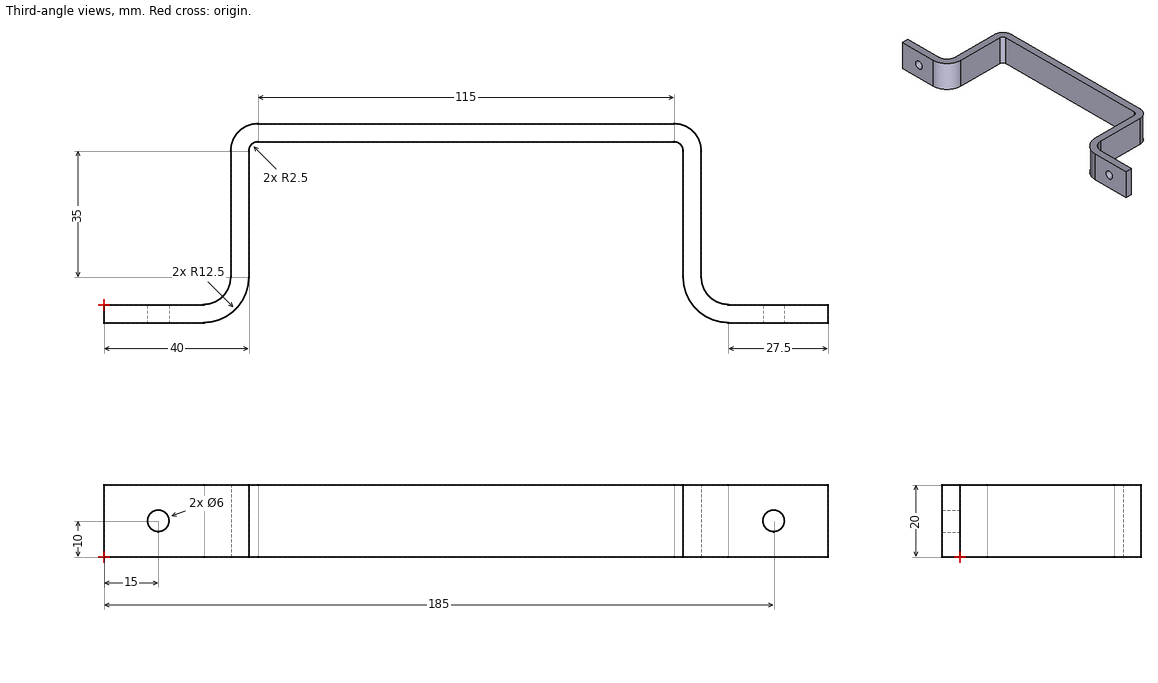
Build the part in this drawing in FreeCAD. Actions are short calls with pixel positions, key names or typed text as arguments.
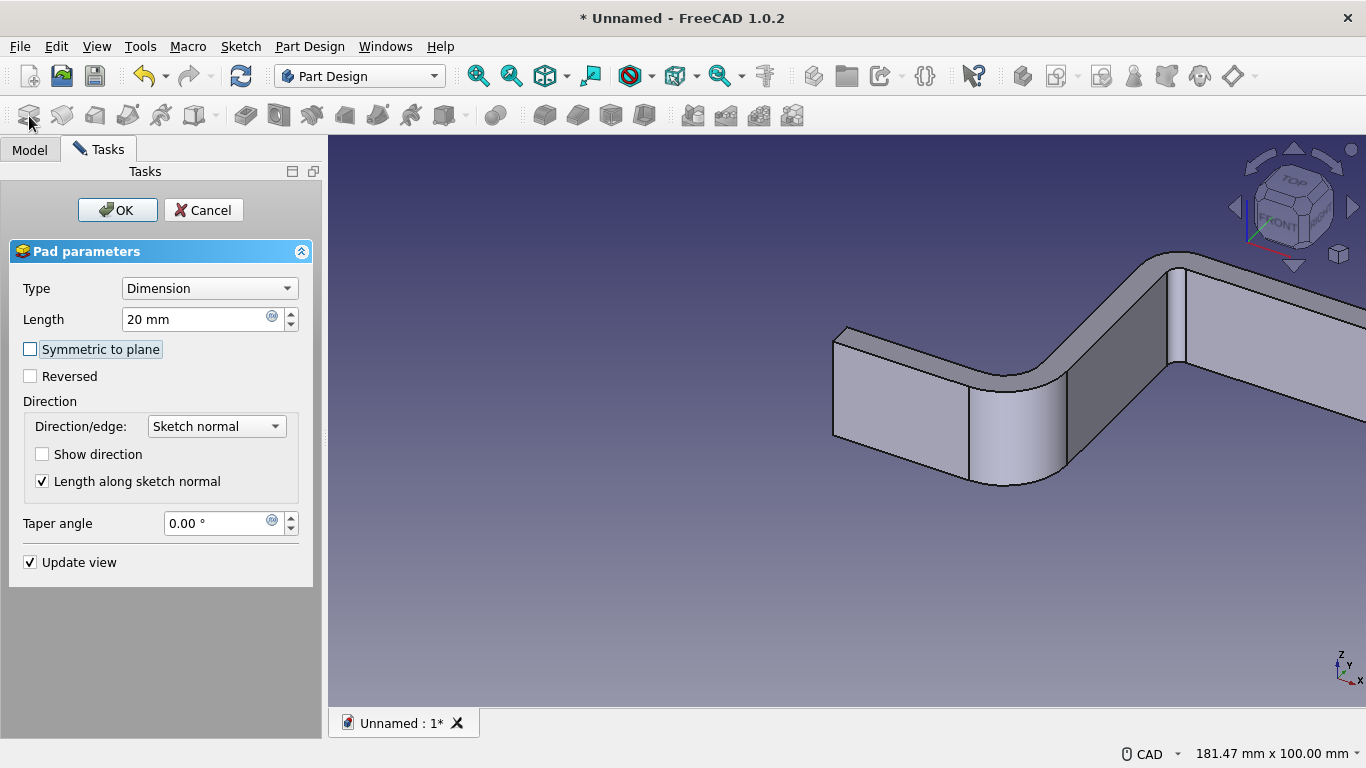
click(118, 210)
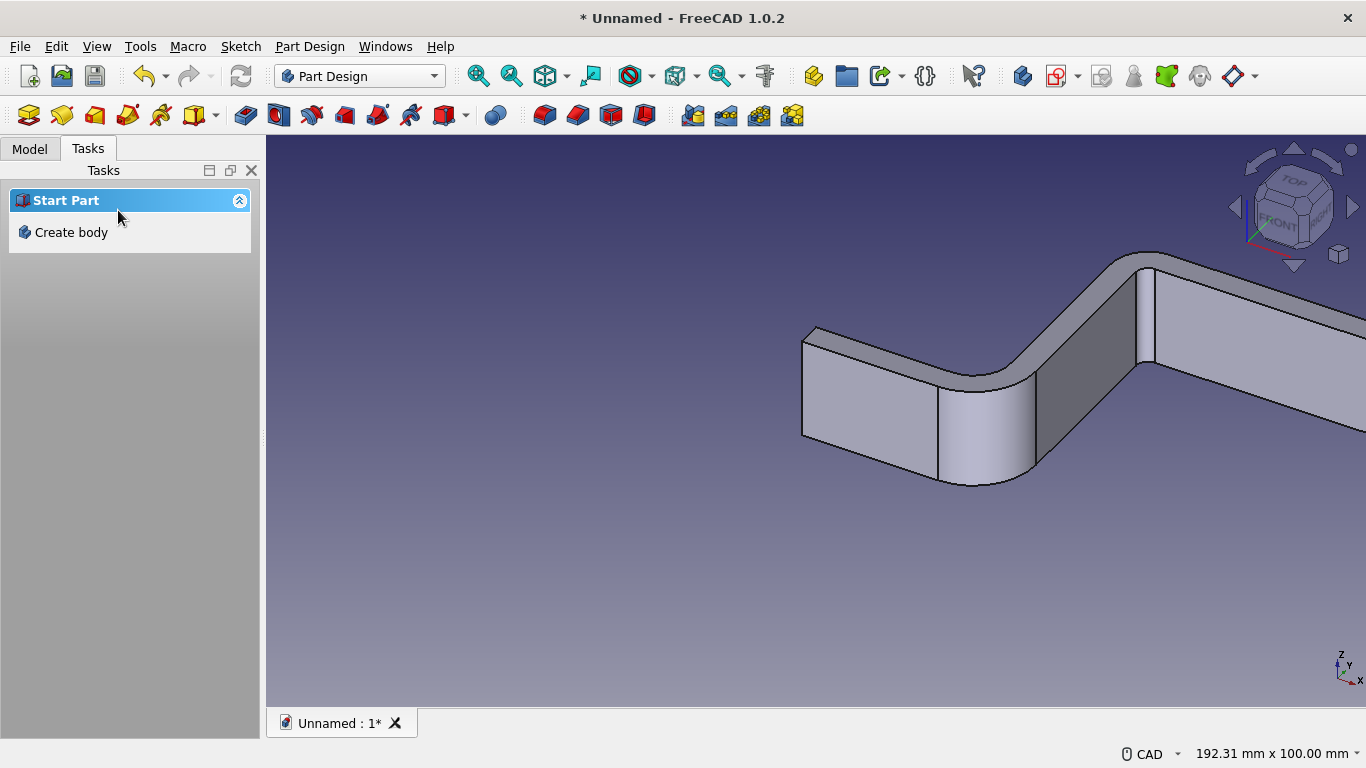
key(v)
key(f)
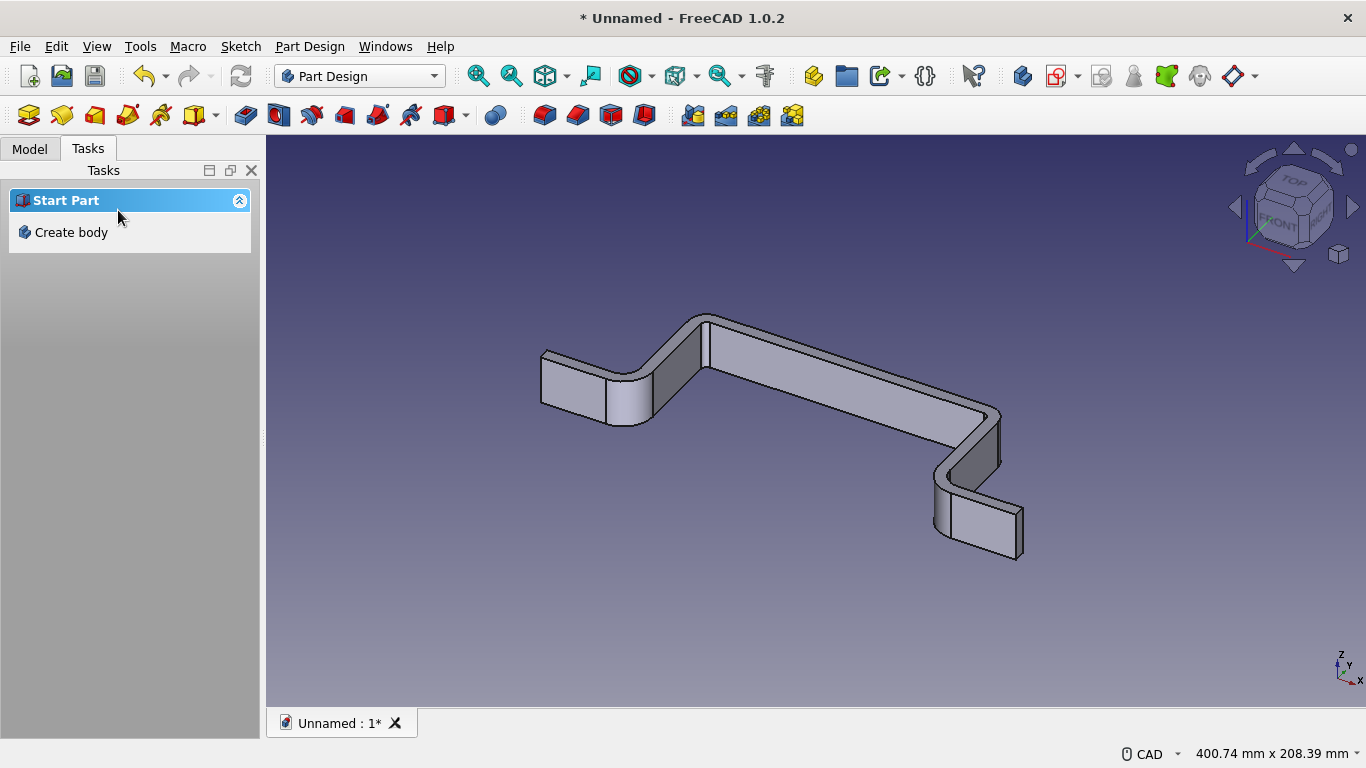
click(573, 390)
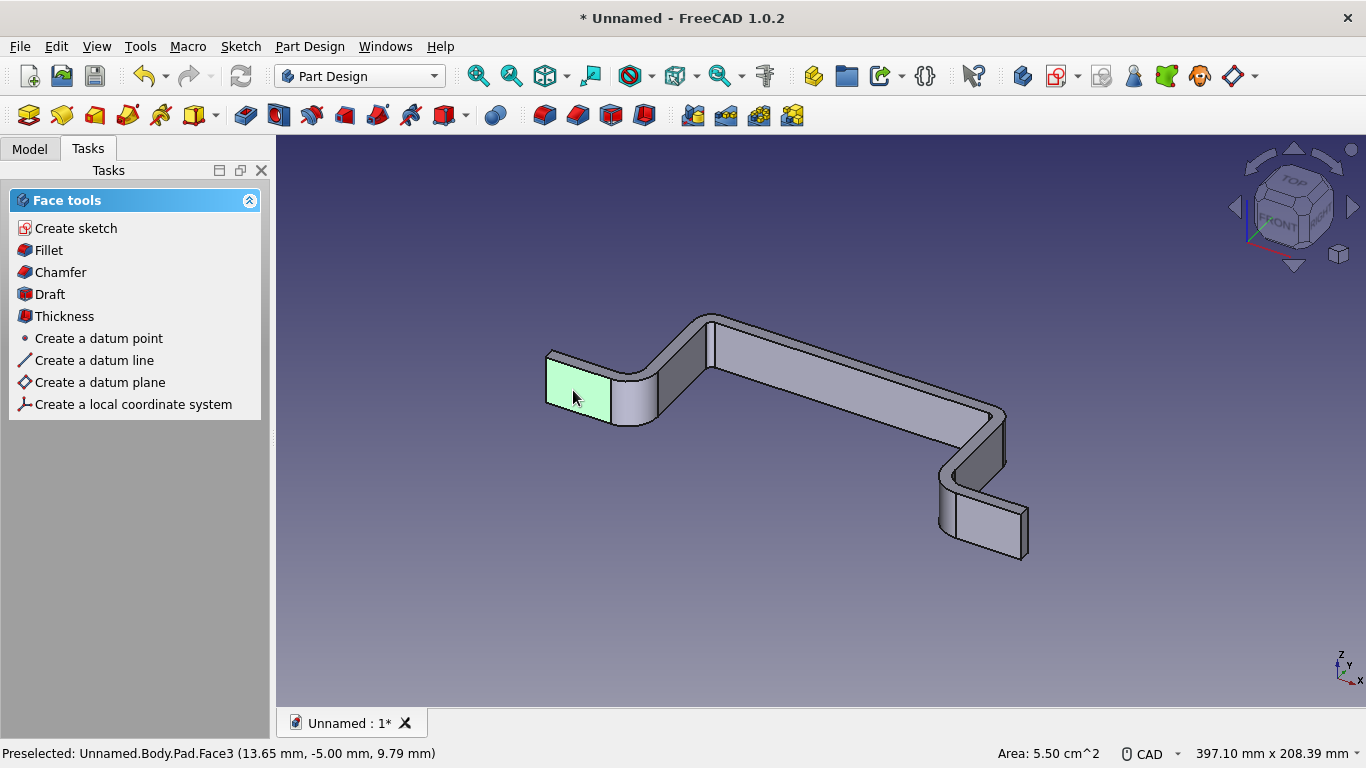
click(1056, 76)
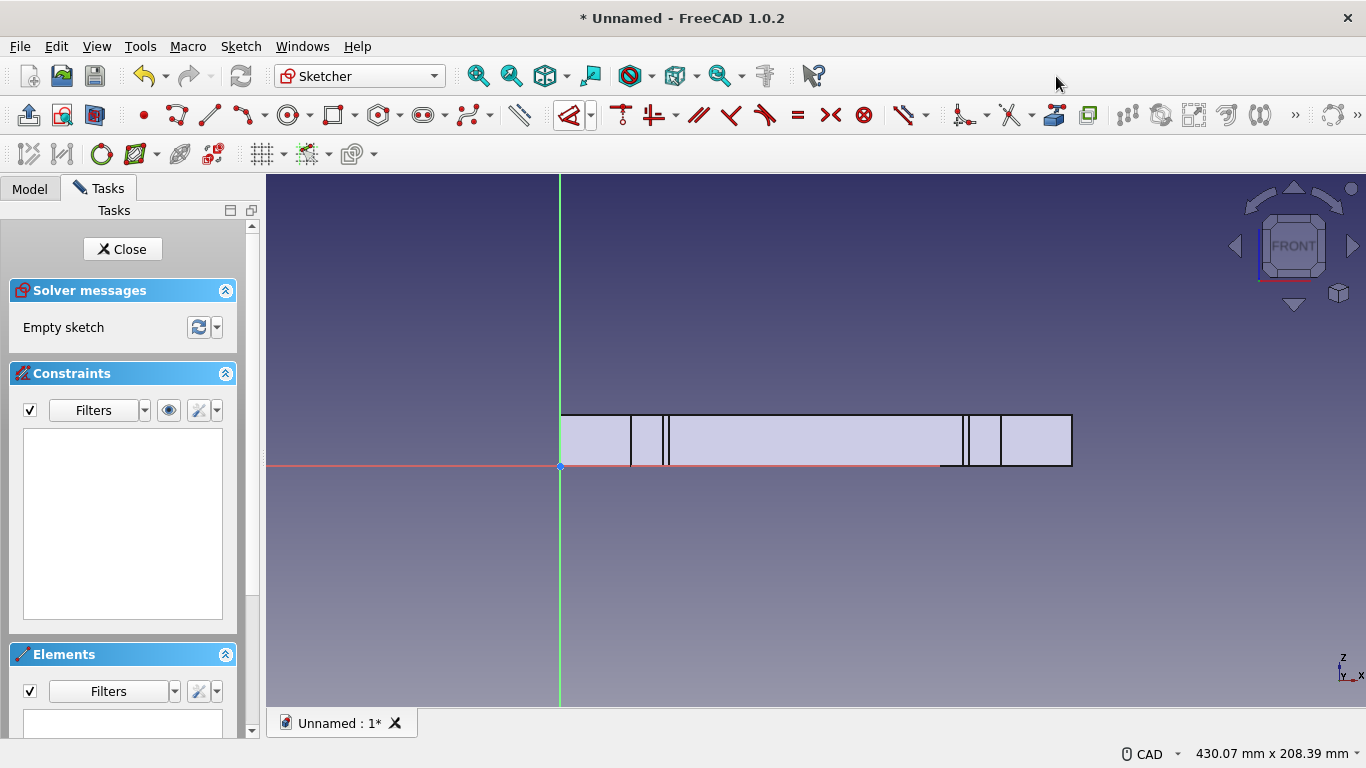
click(288, 116)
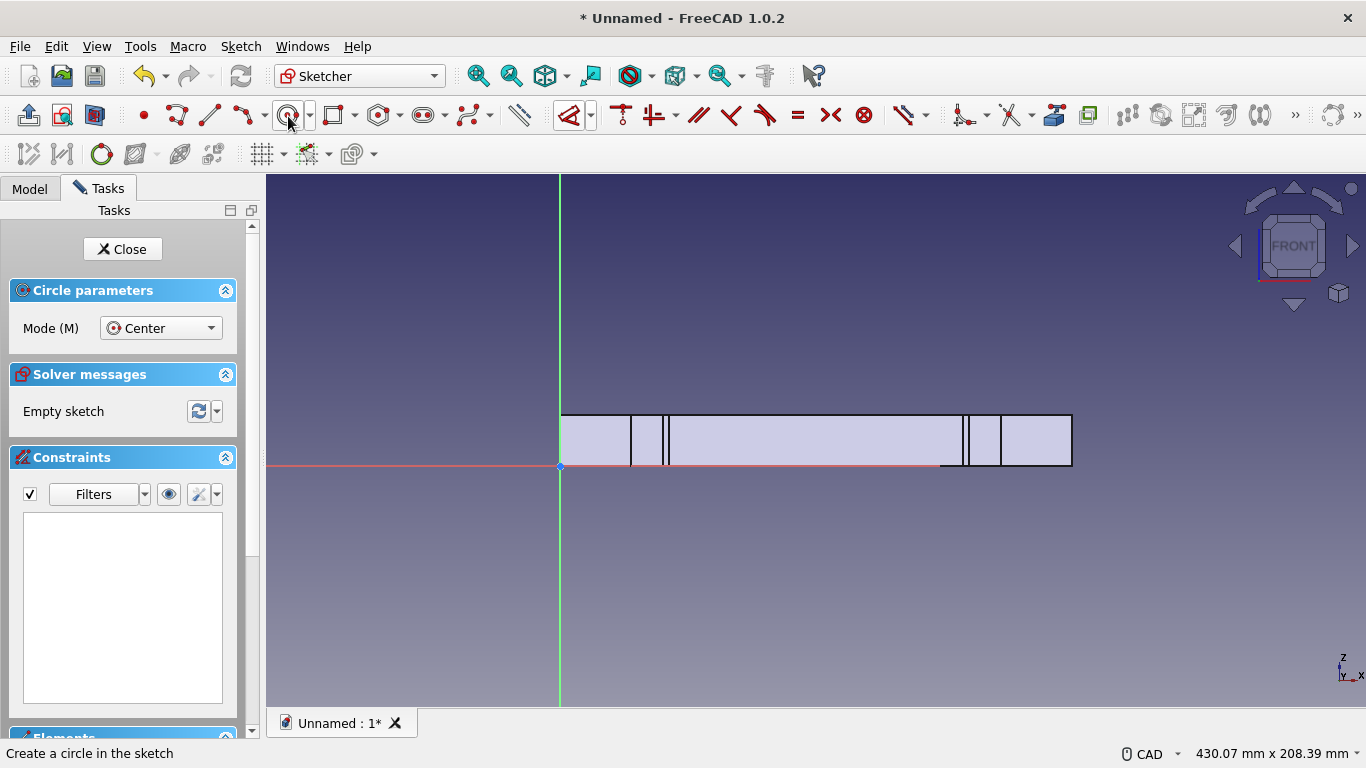
scroll(599, 440, up, 6)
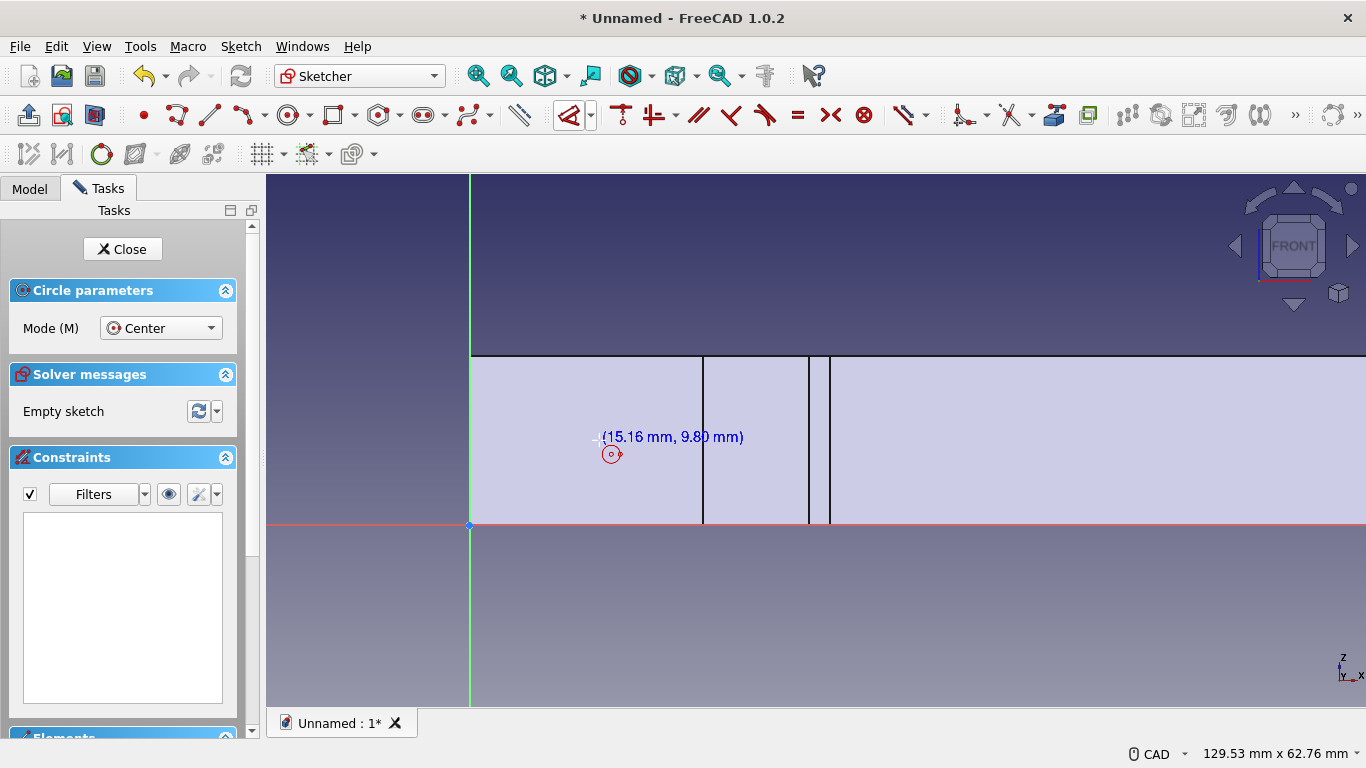
click(597, 440)
click(615, 422)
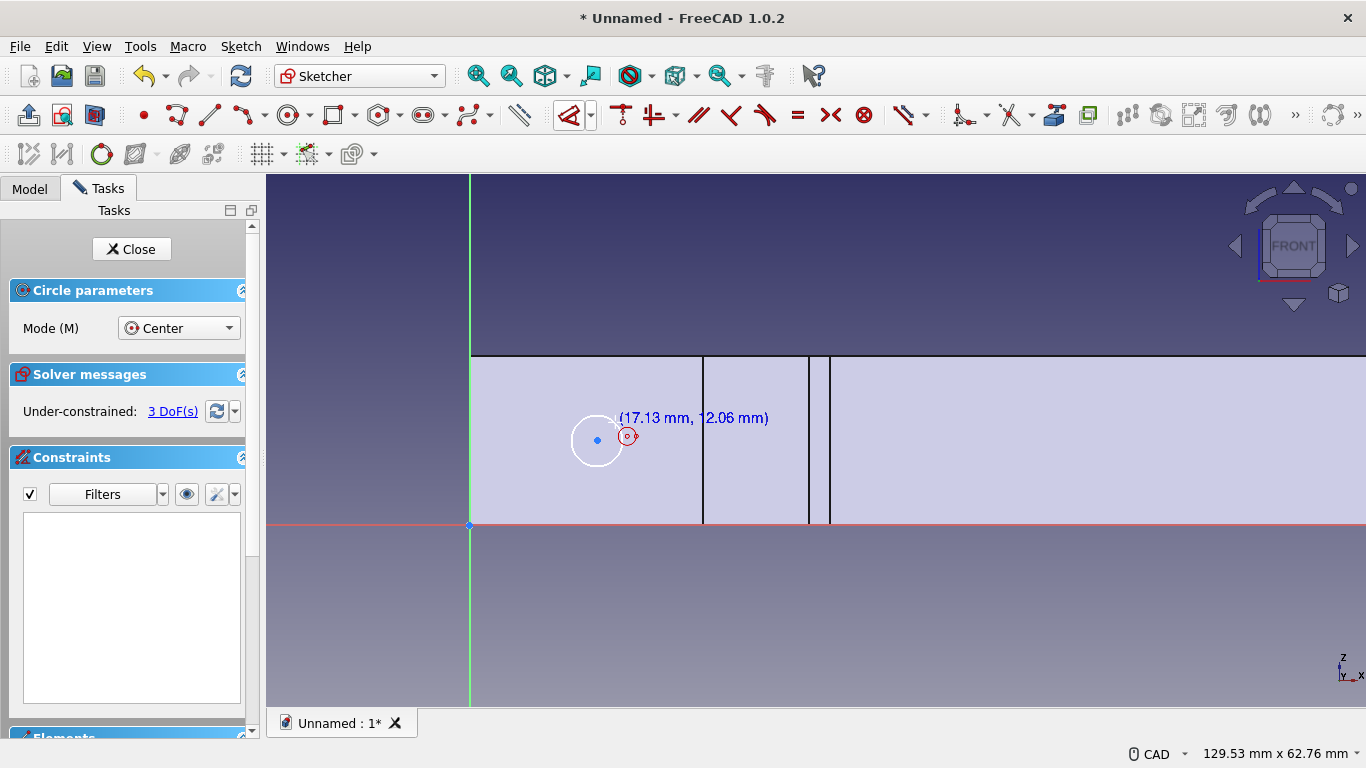
scroll(445, 423, down, 5)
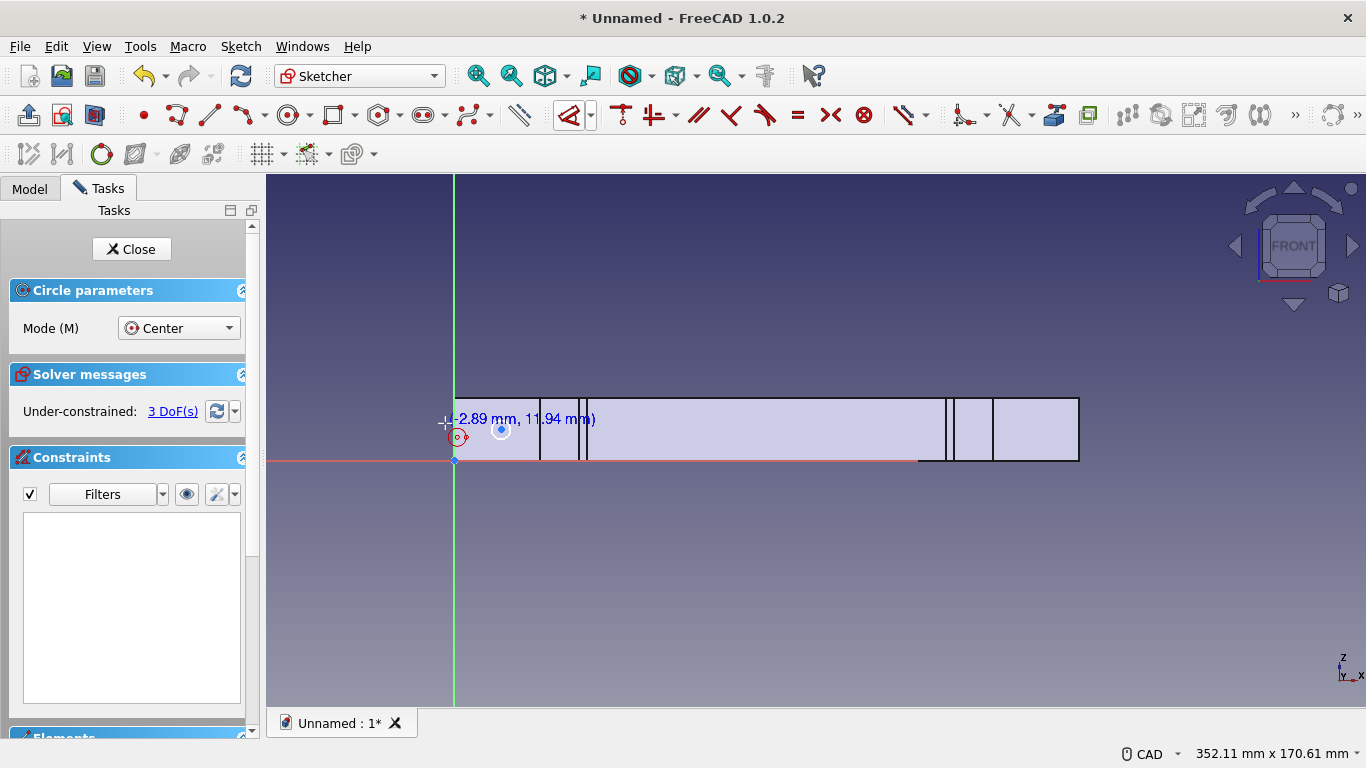
scroll(1032, 430, up, 5)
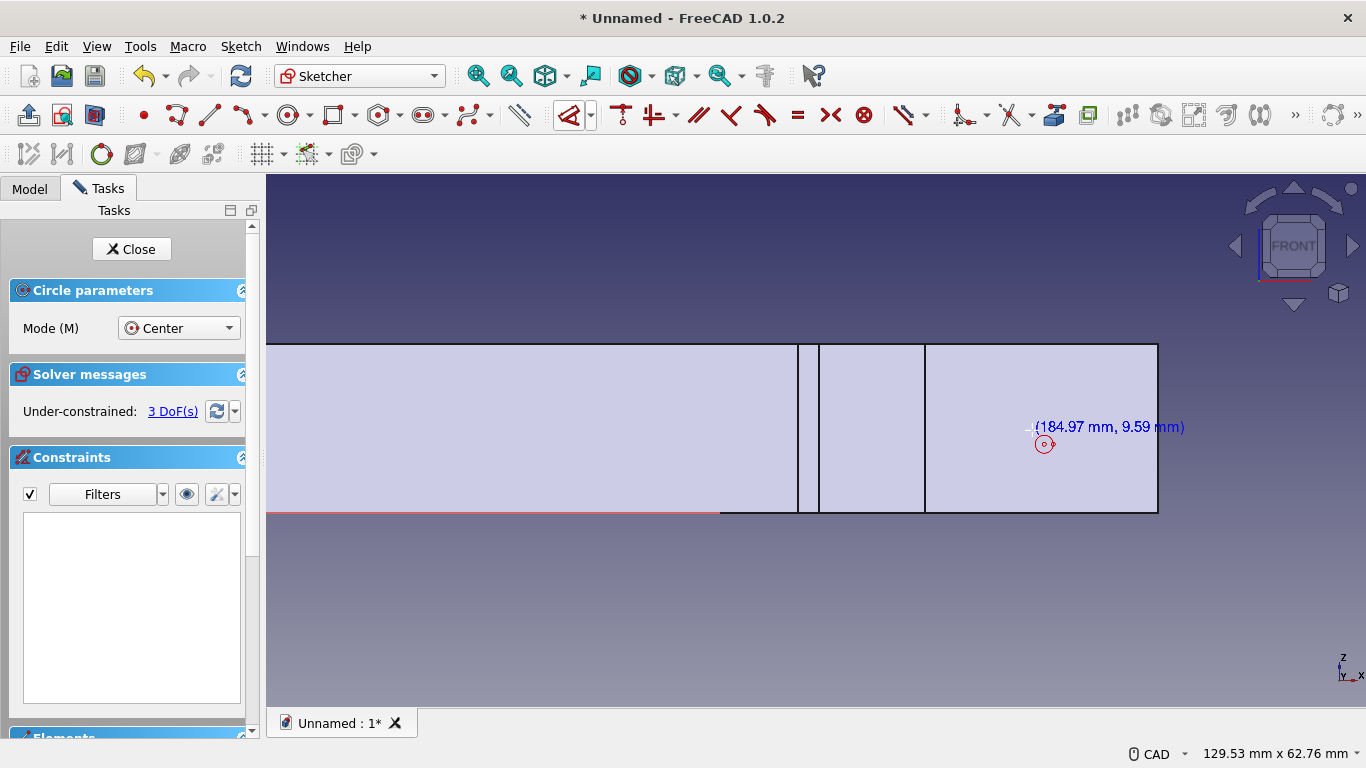
click(1031, 428)
click(1049, 410)
key(Escape)